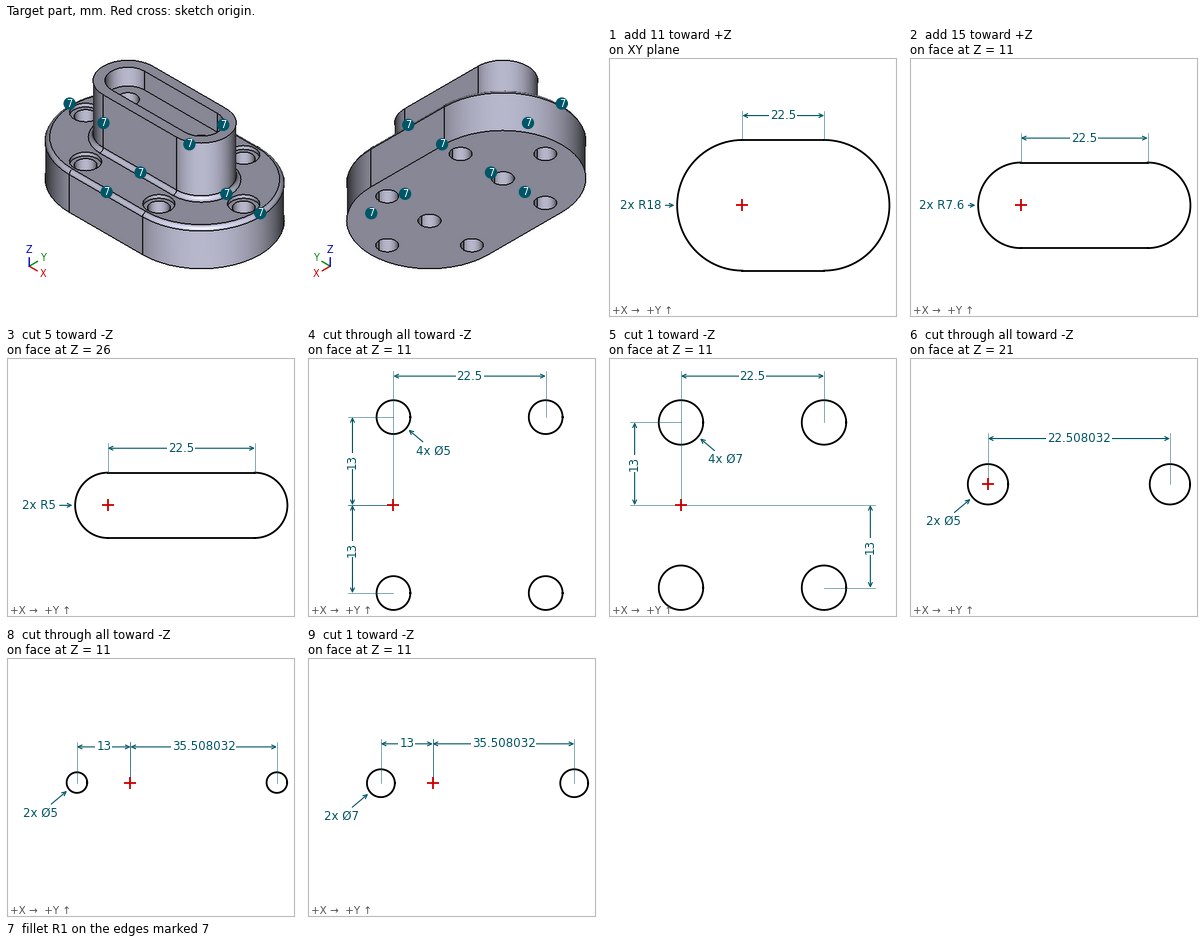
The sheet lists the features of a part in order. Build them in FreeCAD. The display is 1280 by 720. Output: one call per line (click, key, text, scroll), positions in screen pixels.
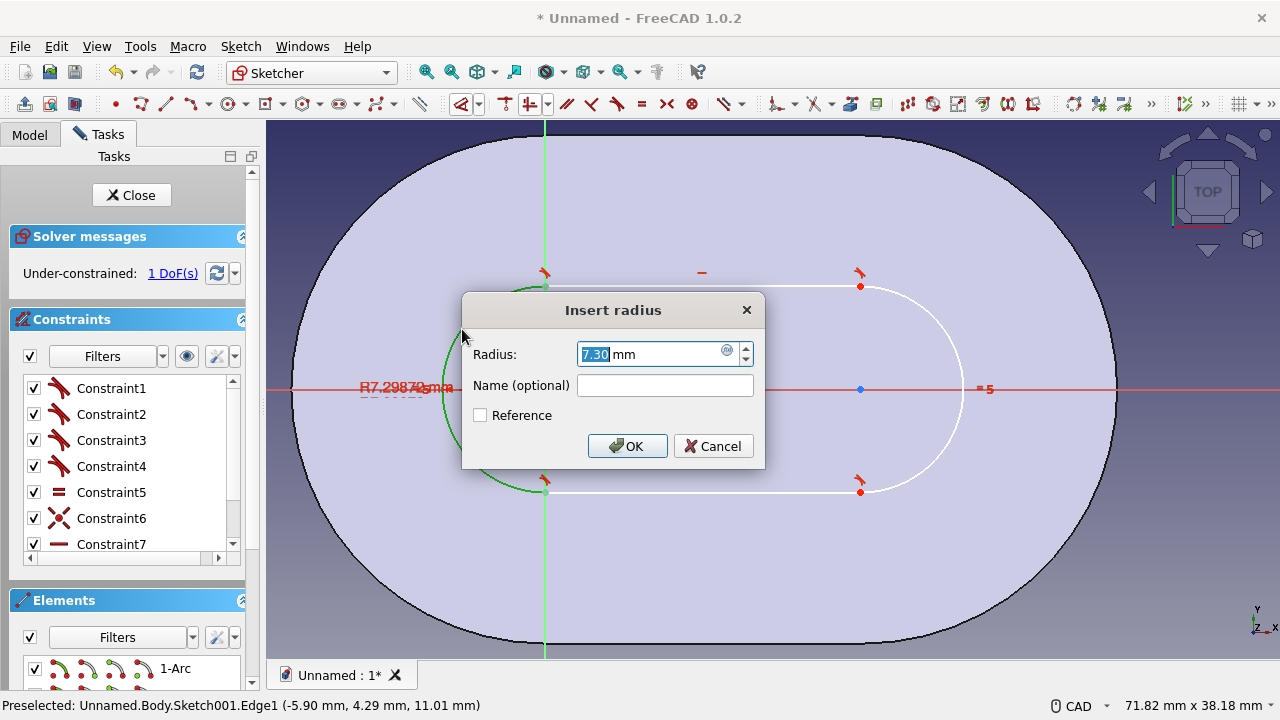
text(7.6)
key(Return)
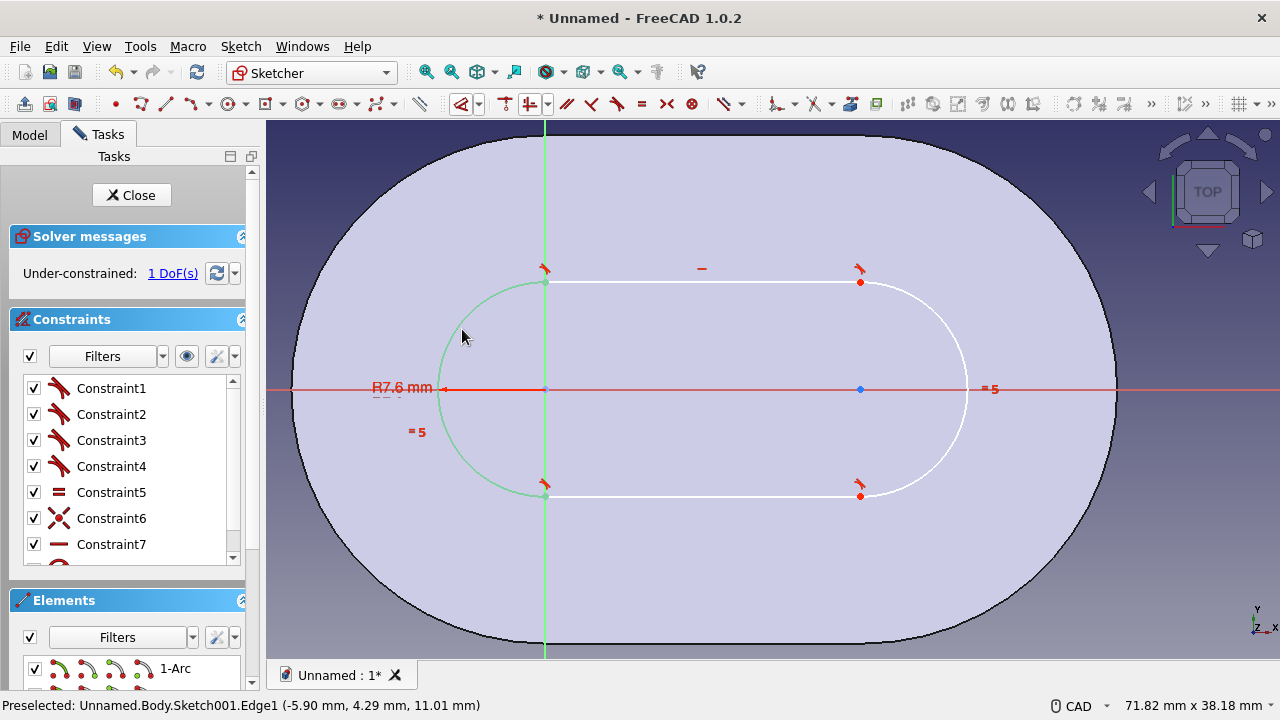
click(640, 282)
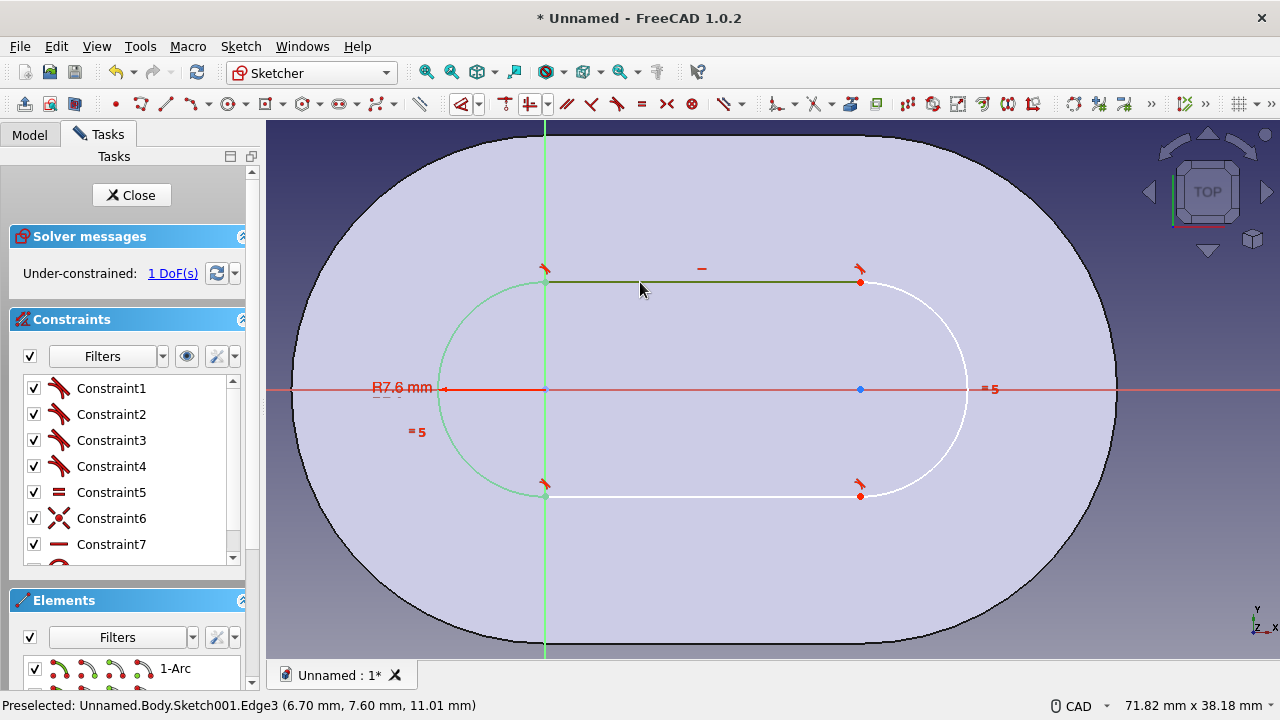
key(l)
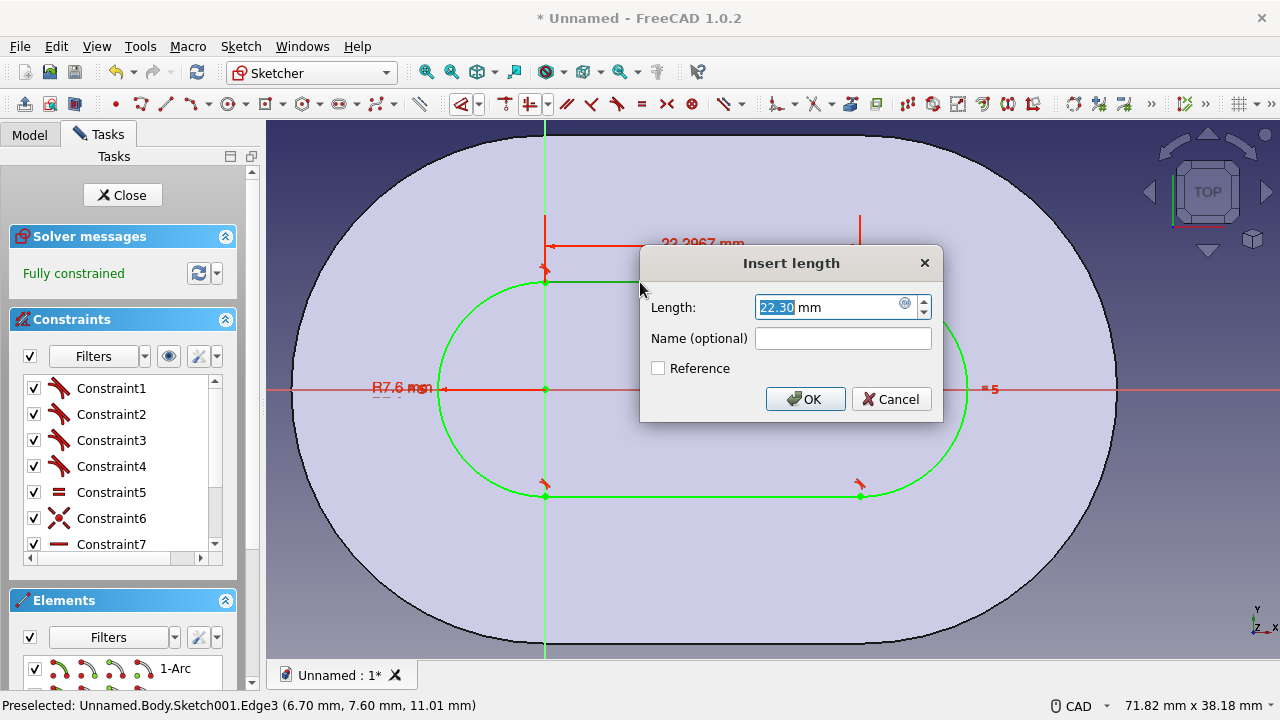
text(22.5)
key(Return)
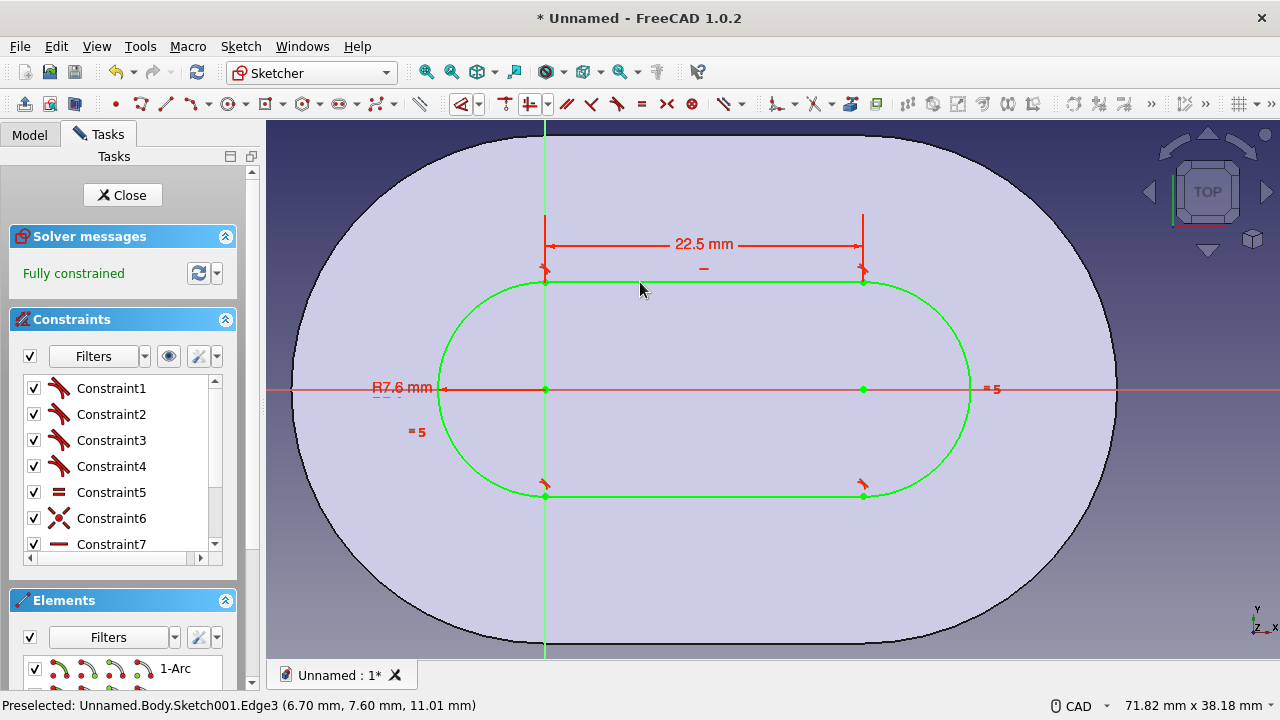
click(123, 195)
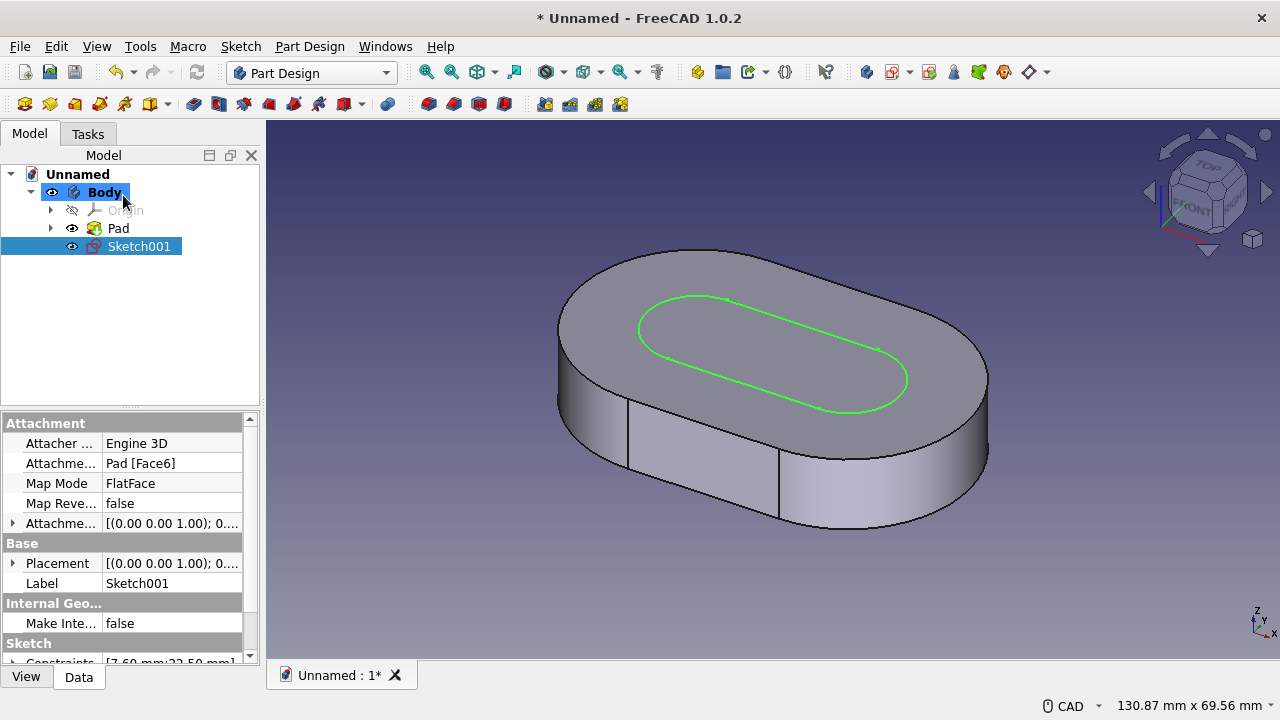
click(25, 104)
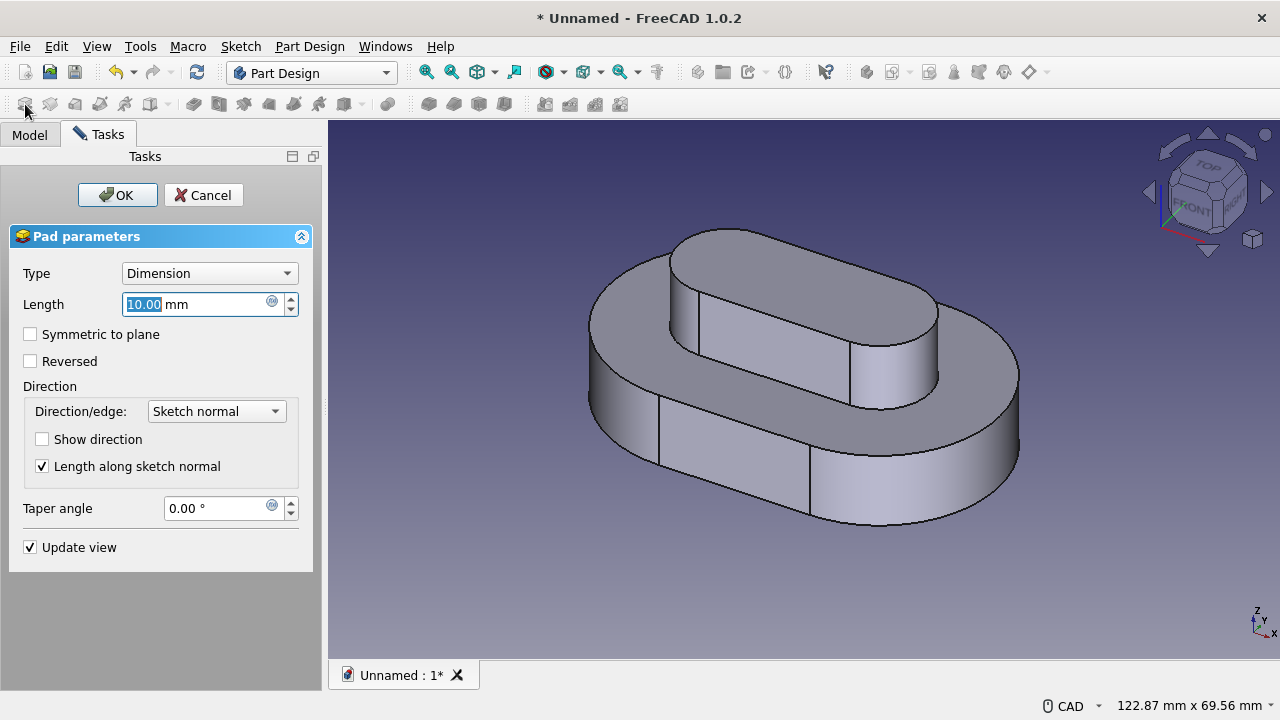
text(15)
key(Tab)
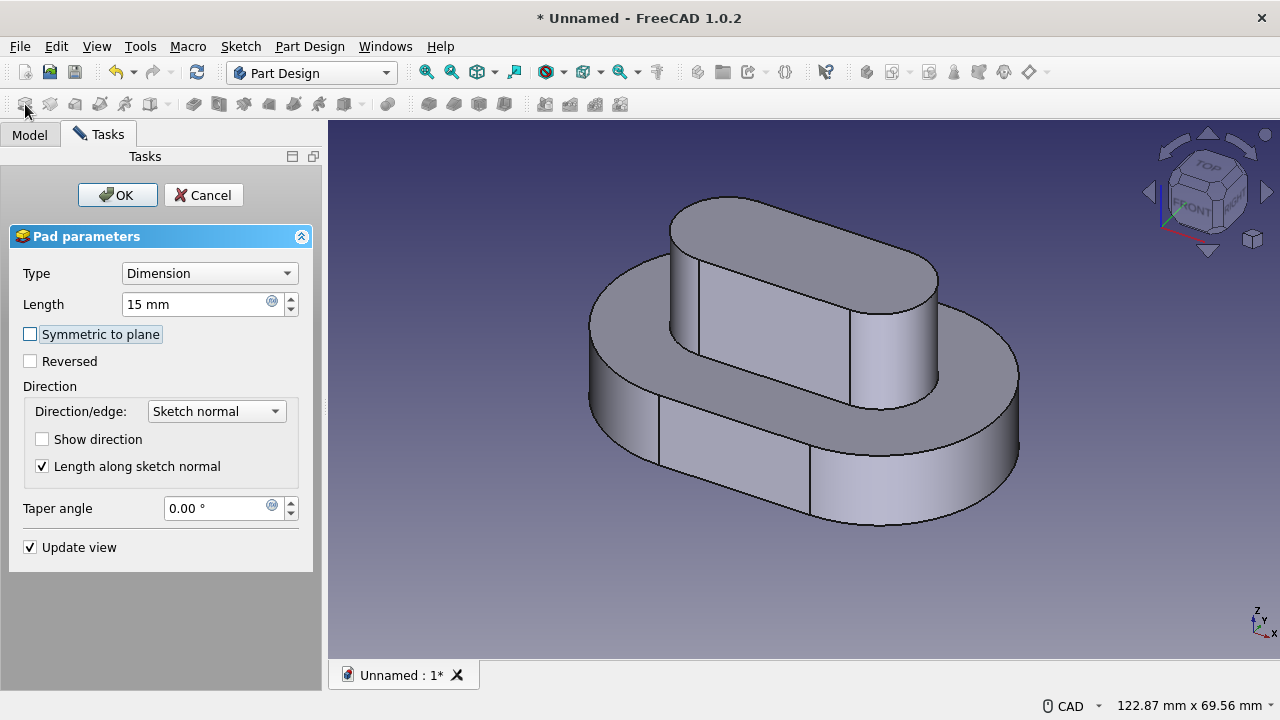
click(118, 195)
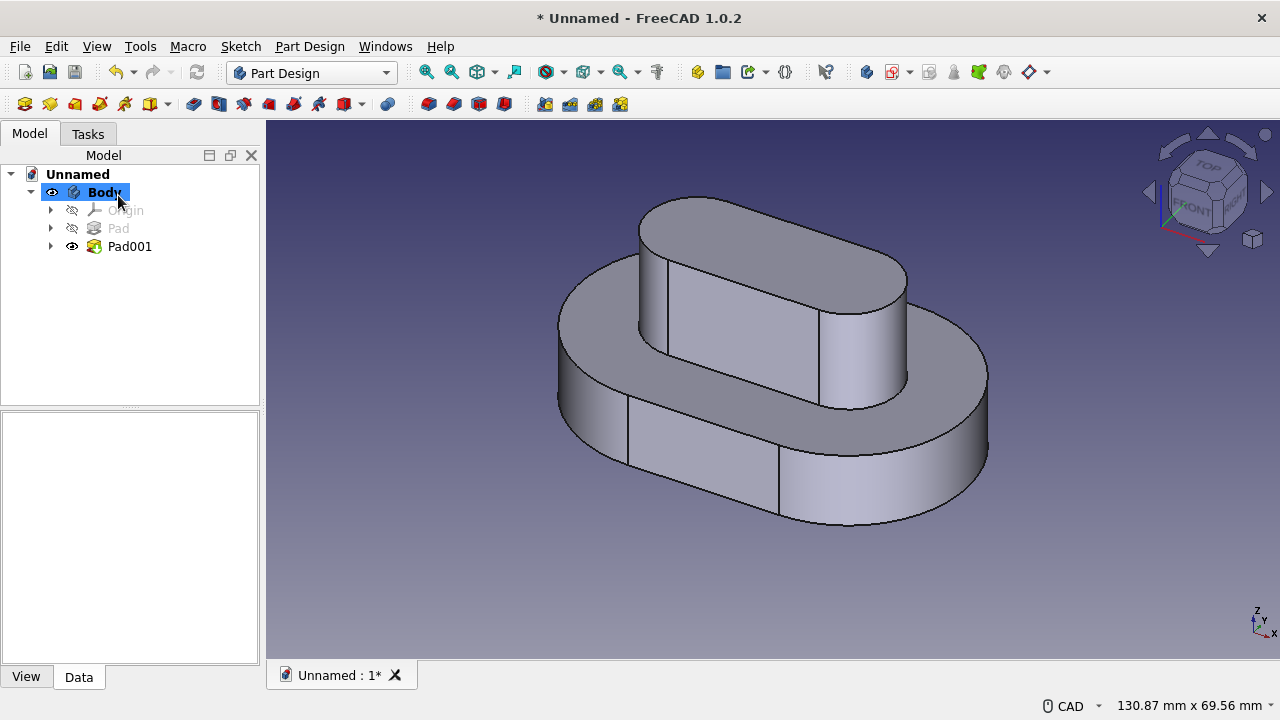
click(845, 279)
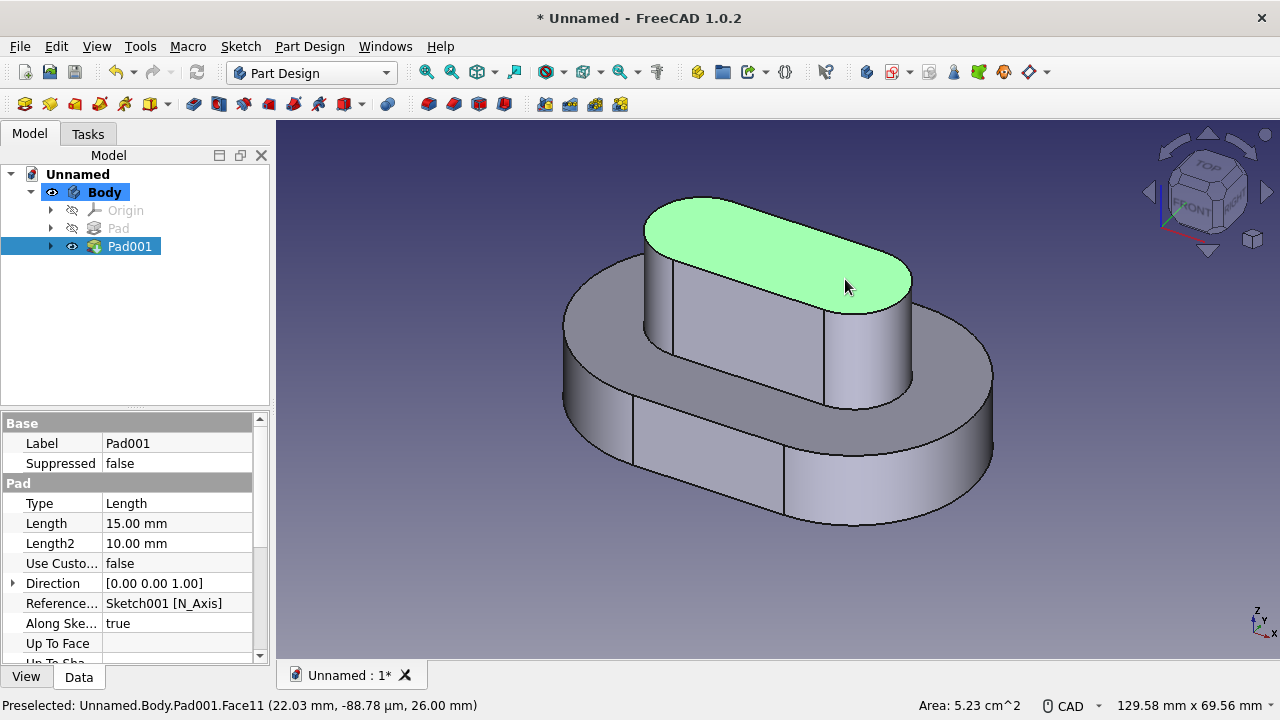
click(892, 72)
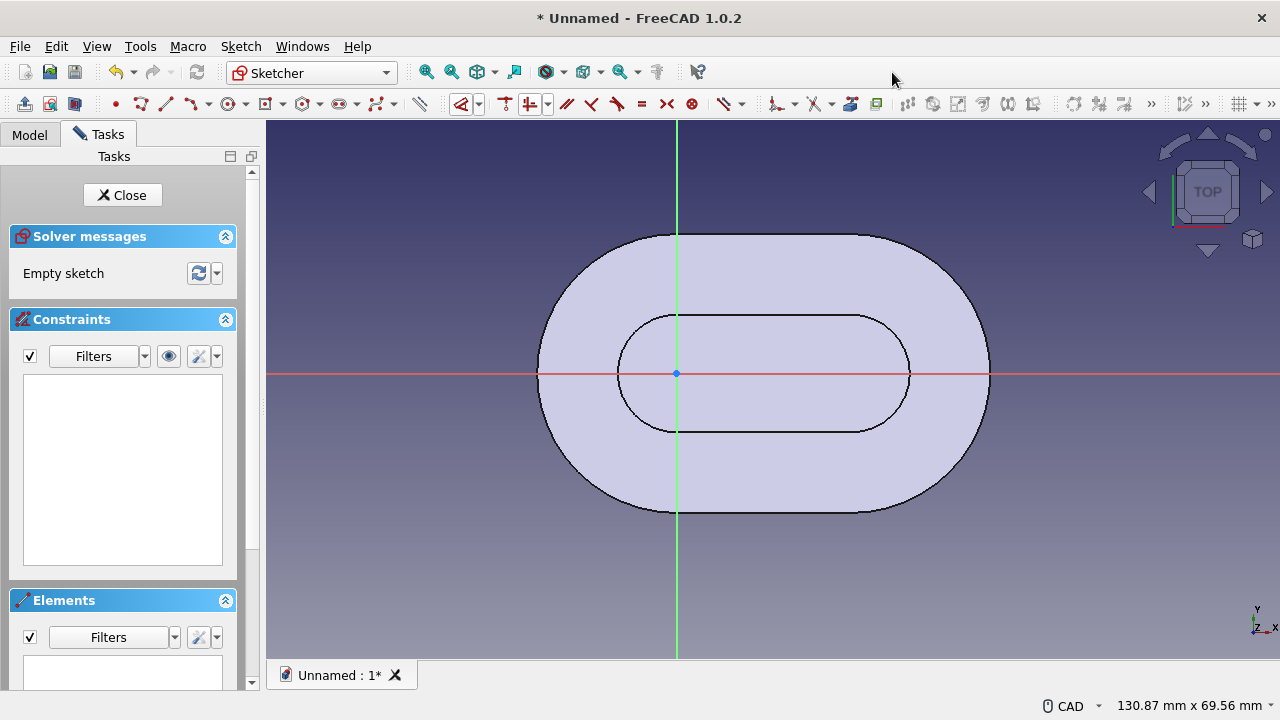
scroll(812, 360, up, 4)